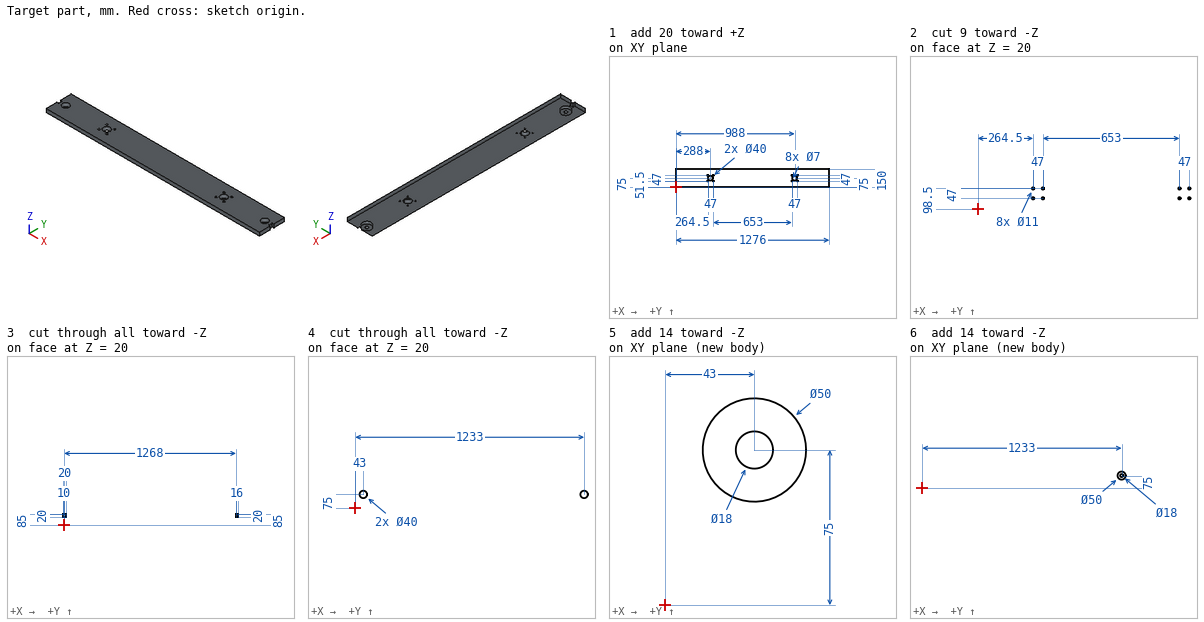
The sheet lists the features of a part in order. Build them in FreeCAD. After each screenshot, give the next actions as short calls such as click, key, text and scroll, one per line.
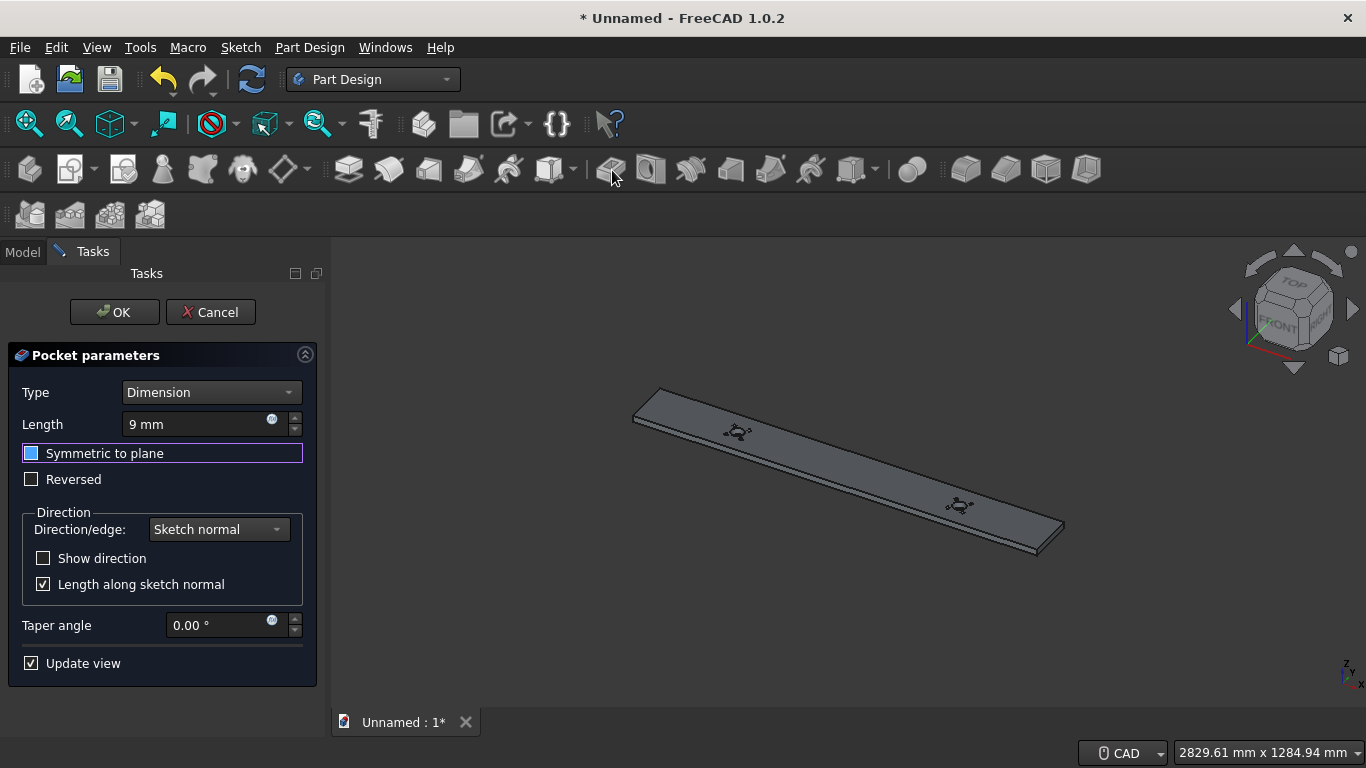
click(115, 312)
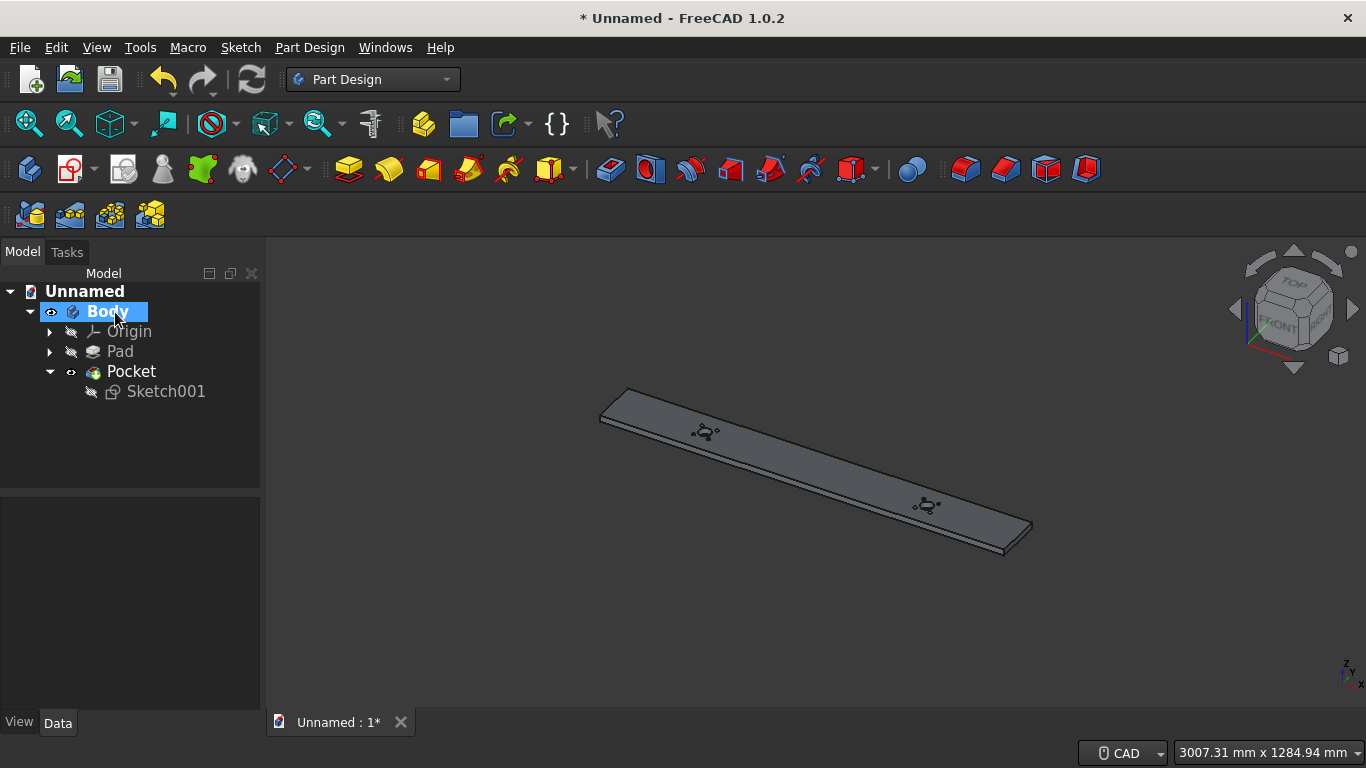
click(30, 124)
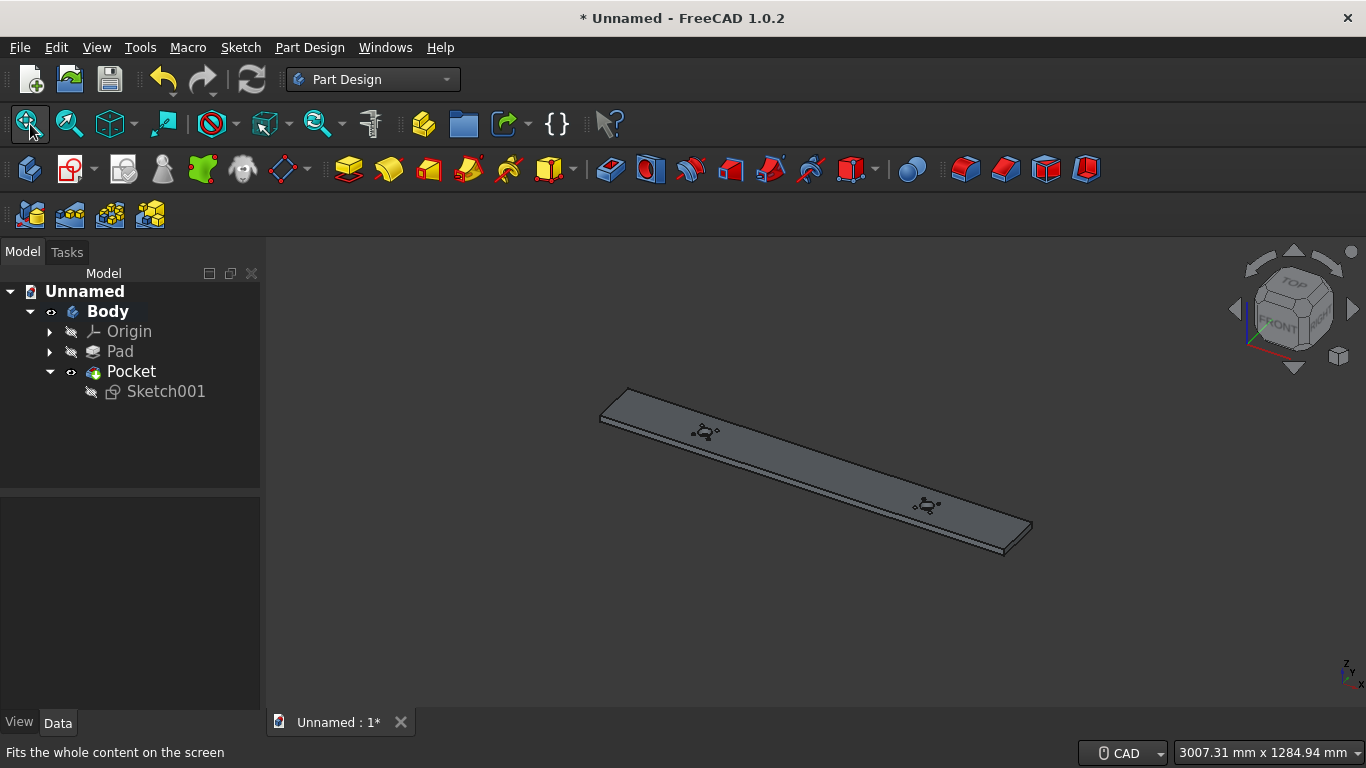
click(989, 525)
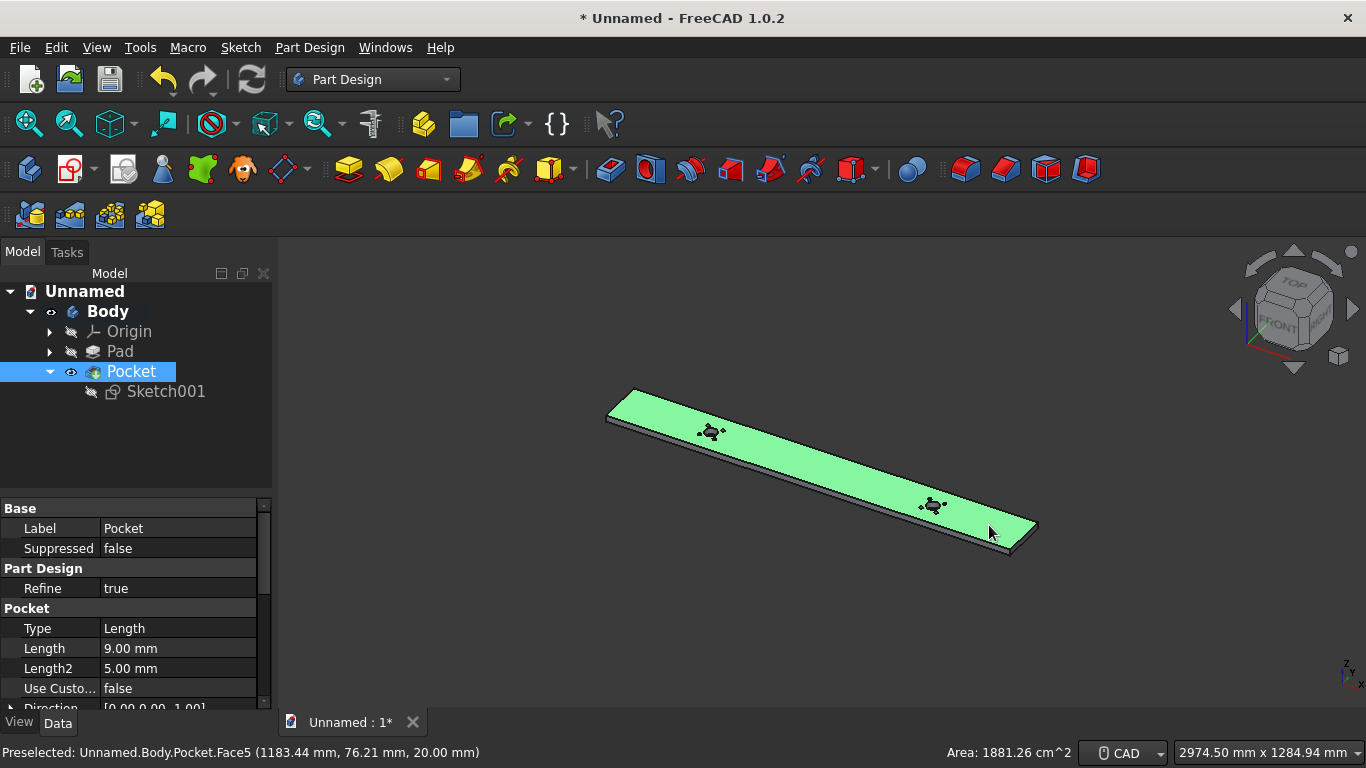
click(70, 170)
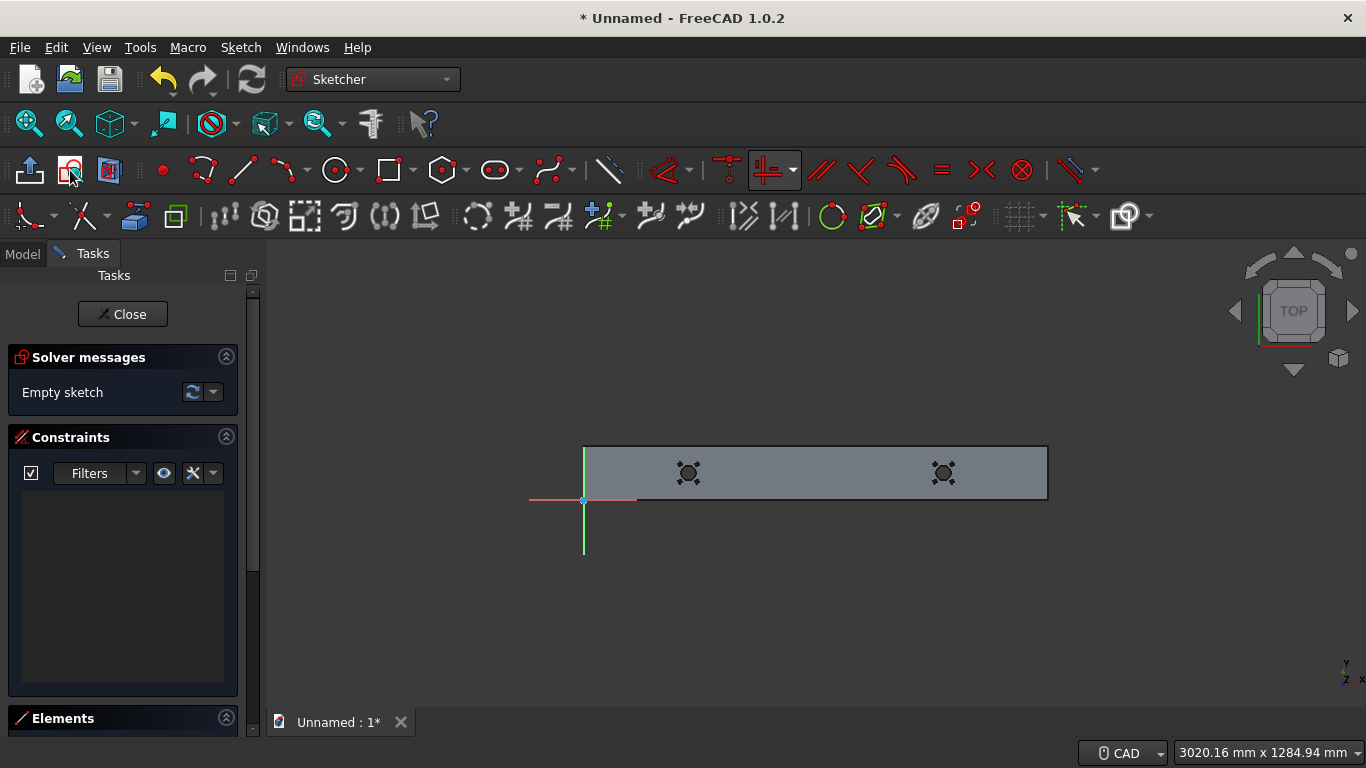
scroll(954, 509, up, 2)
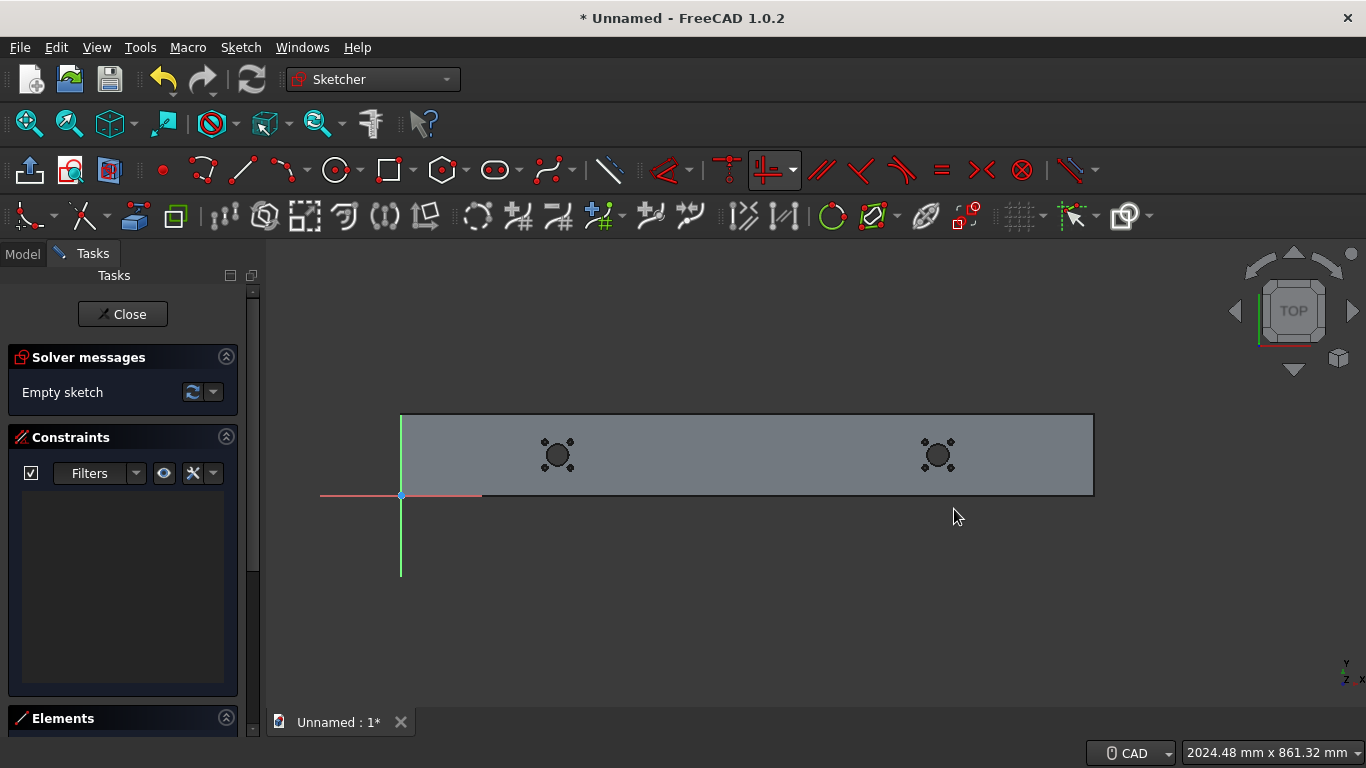
click(390, 170)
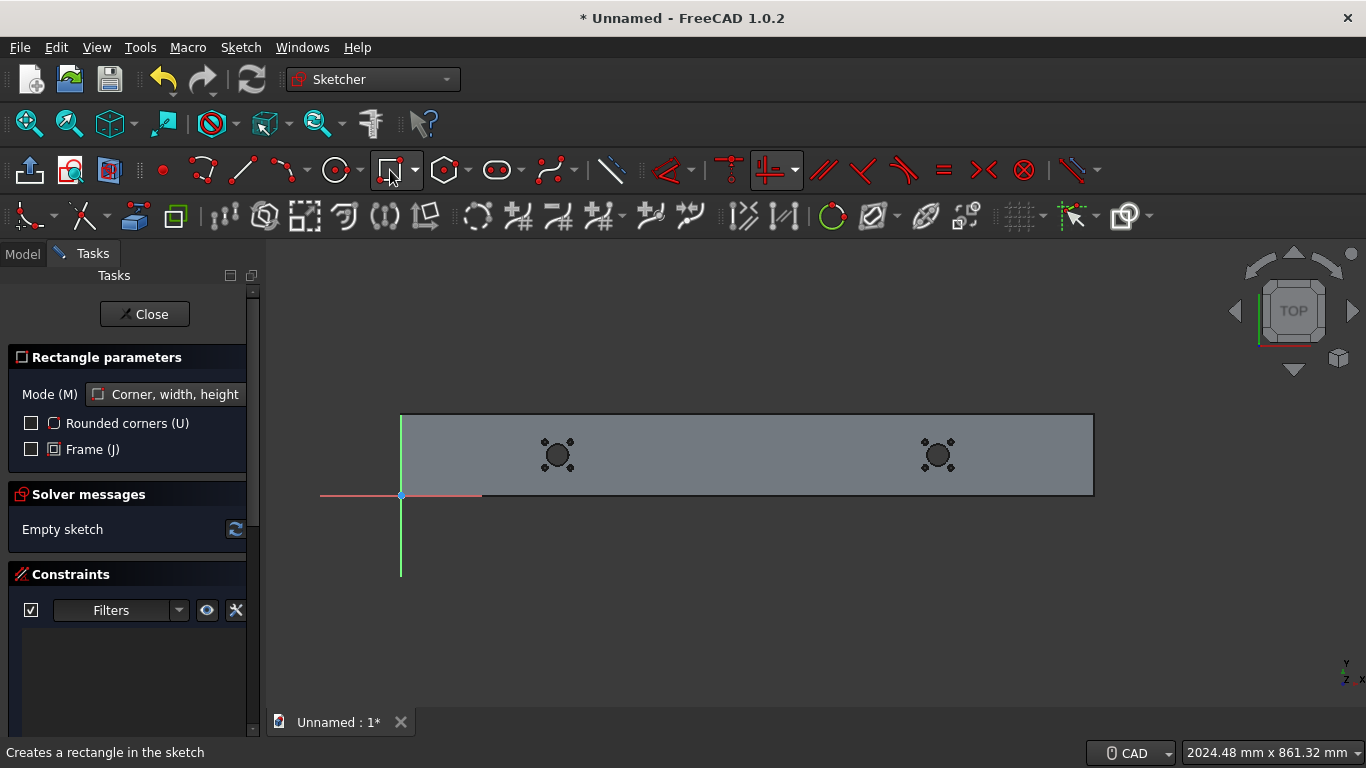
scroll(396, 450, up, 6)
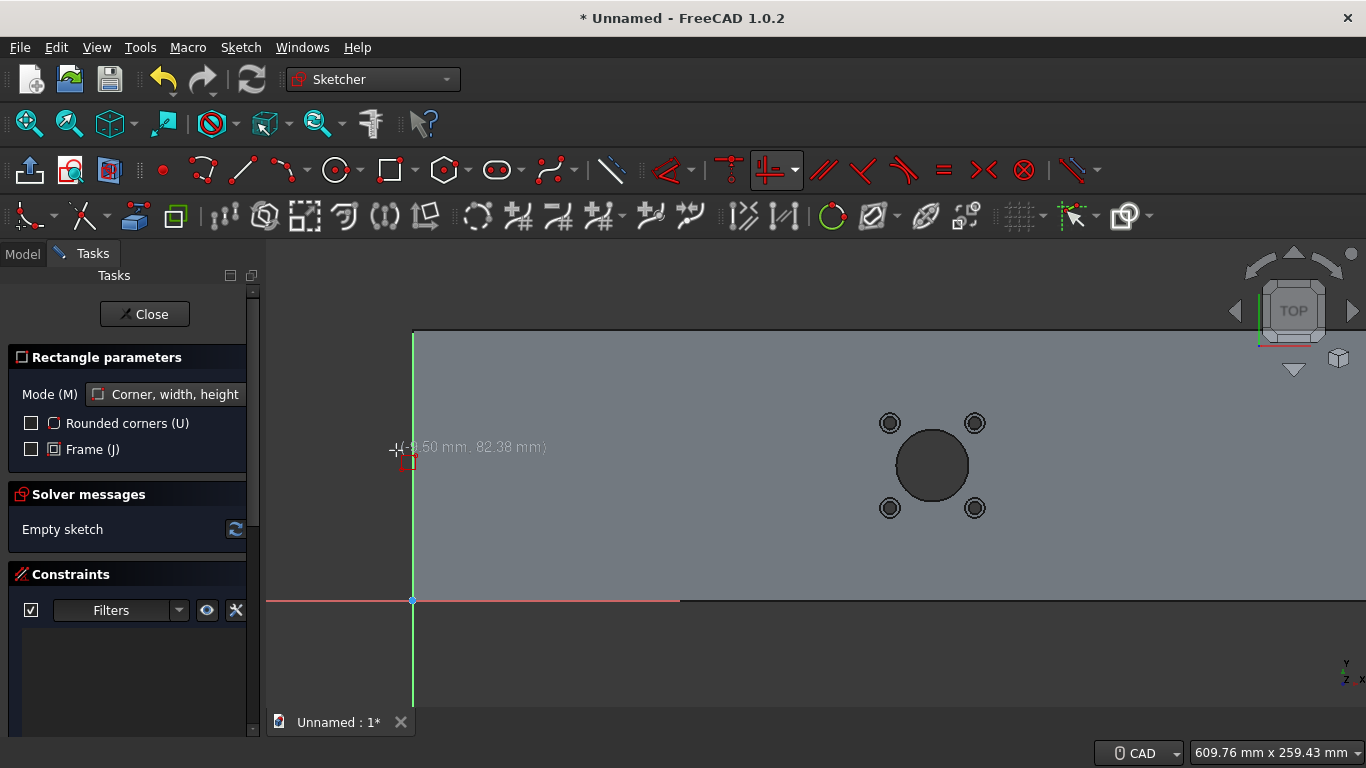
click(395, 448)
move(431, 484)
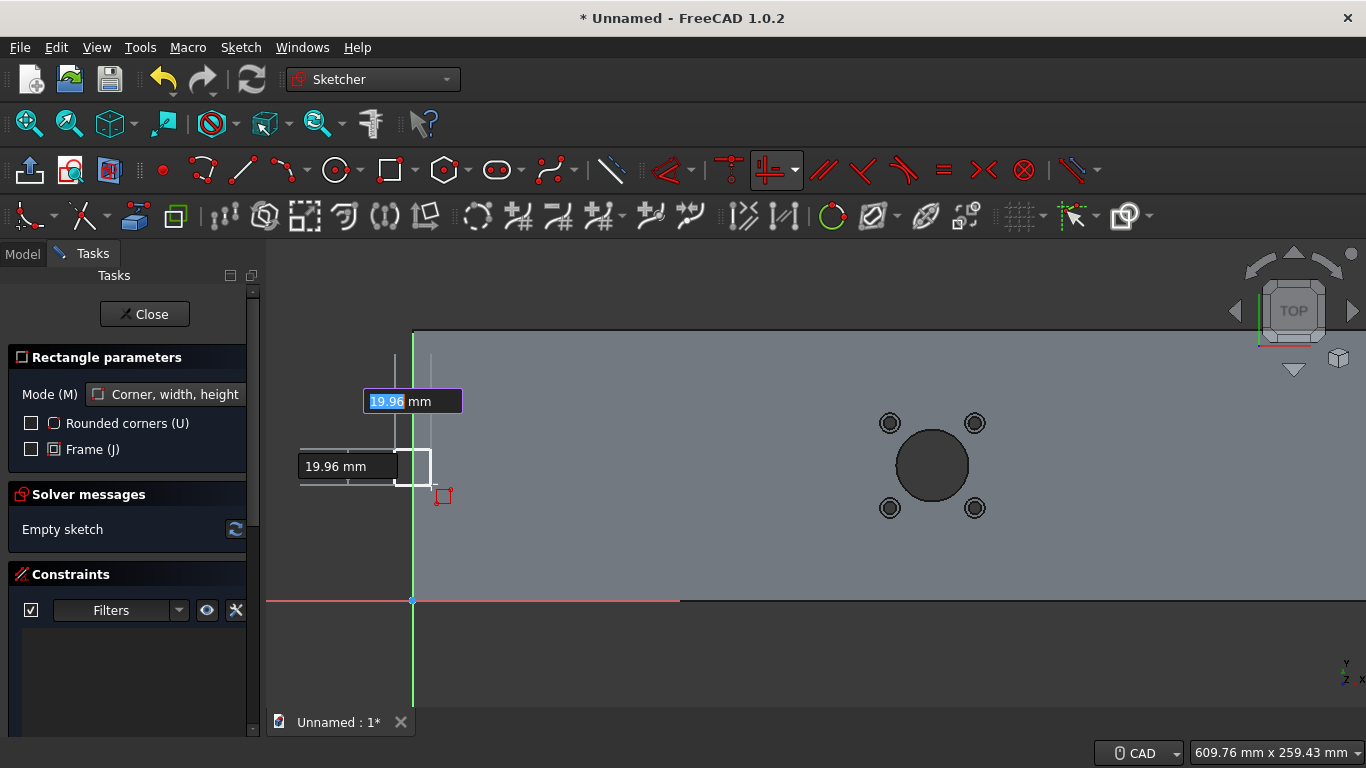
text(20)
key(Tab)
text(20)
key(Return)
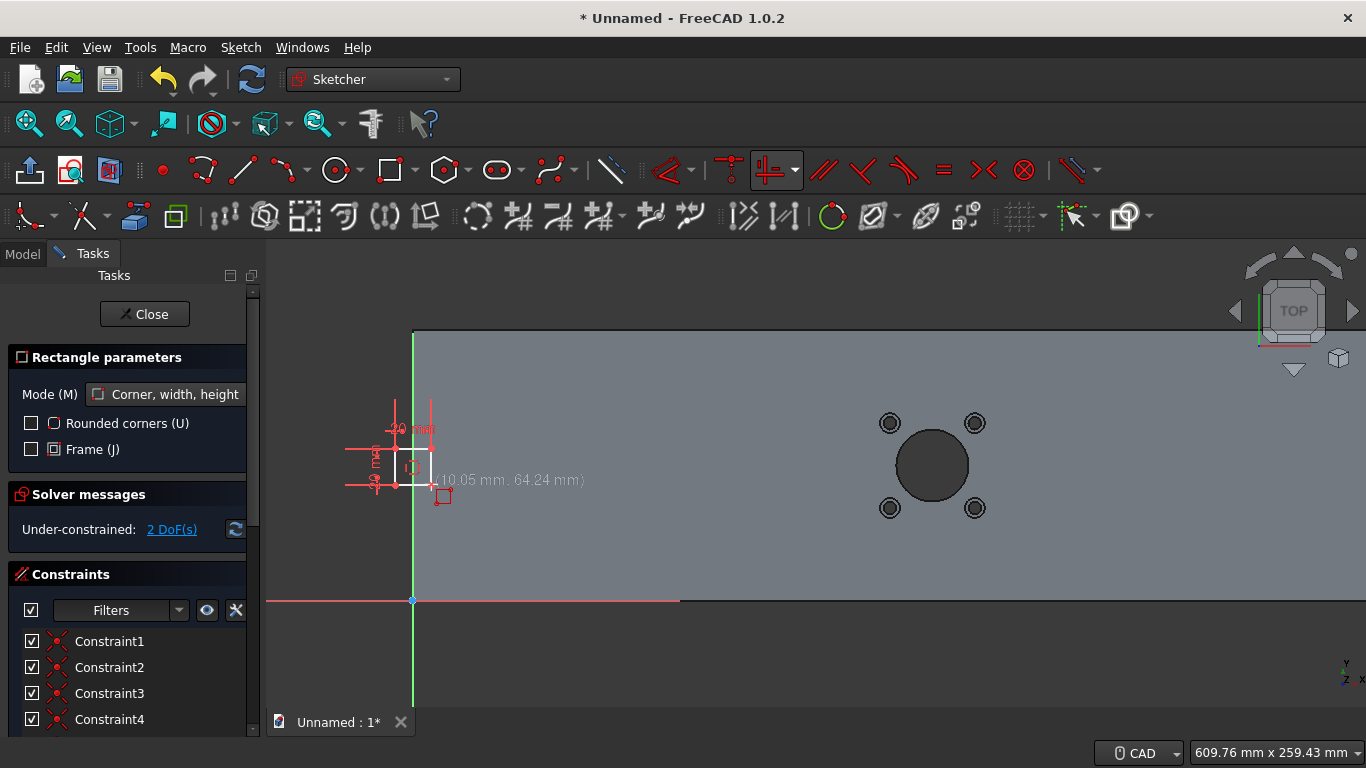
scroll(396, 451, down, 6)